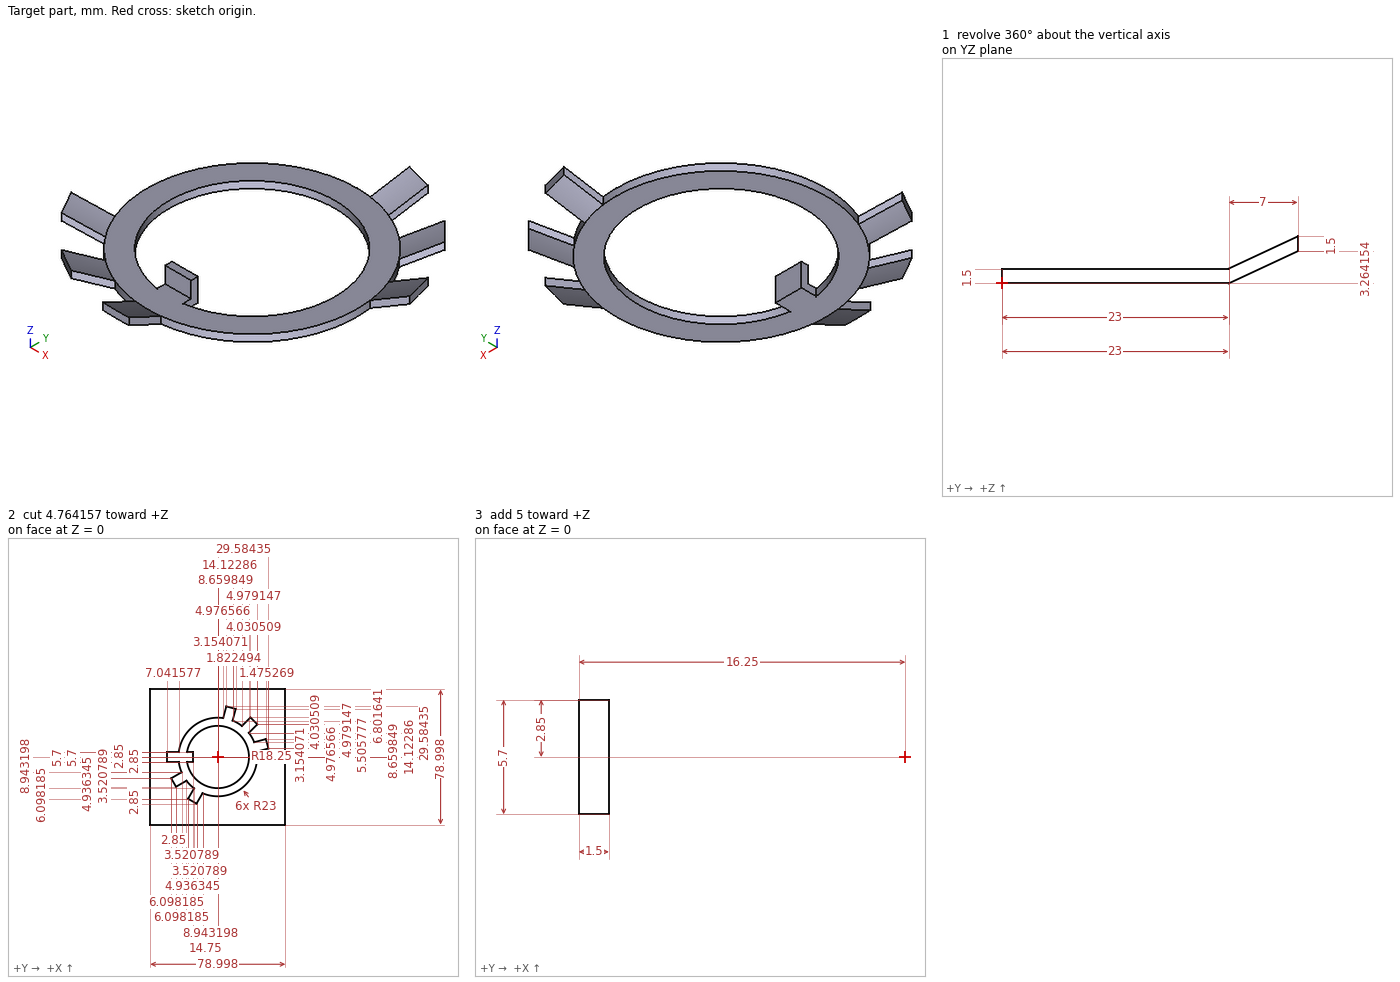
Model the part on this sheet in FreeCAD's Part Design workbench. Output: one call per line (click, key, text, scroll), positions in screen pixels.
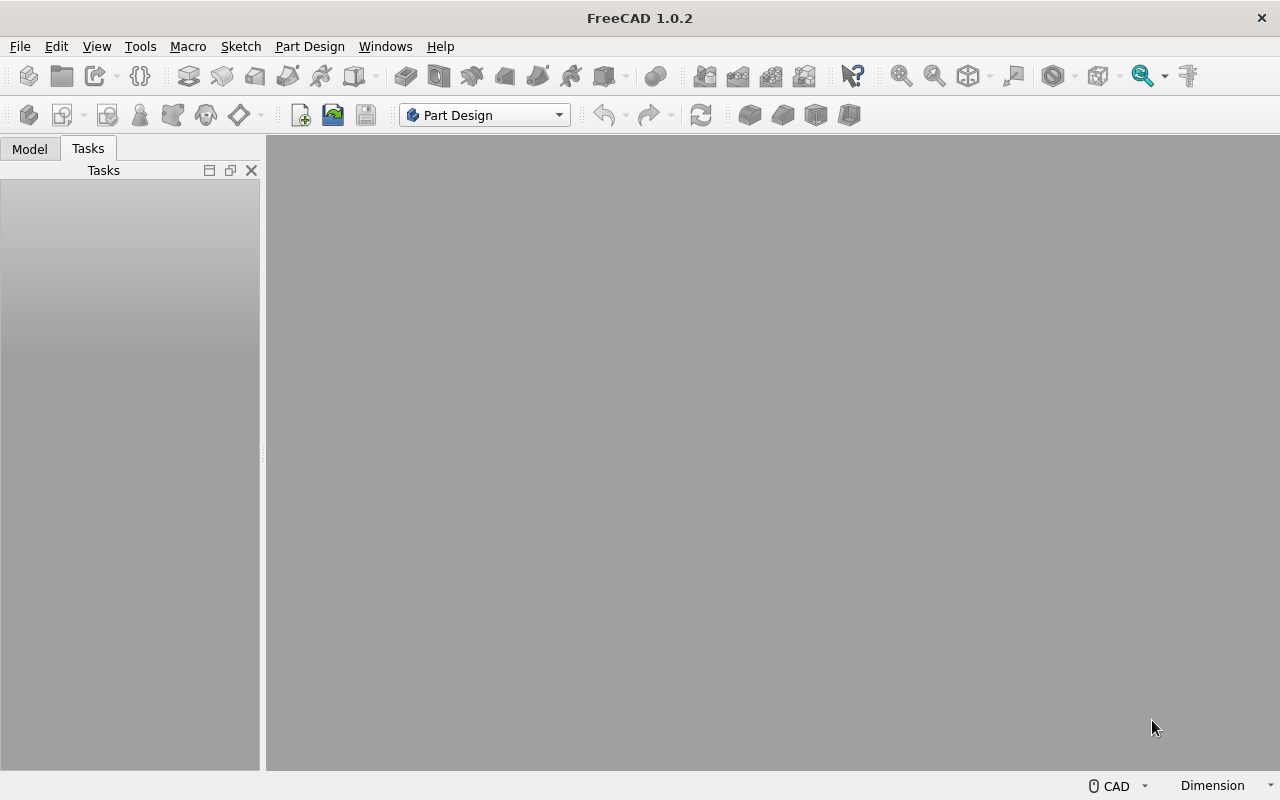
click(300, 116)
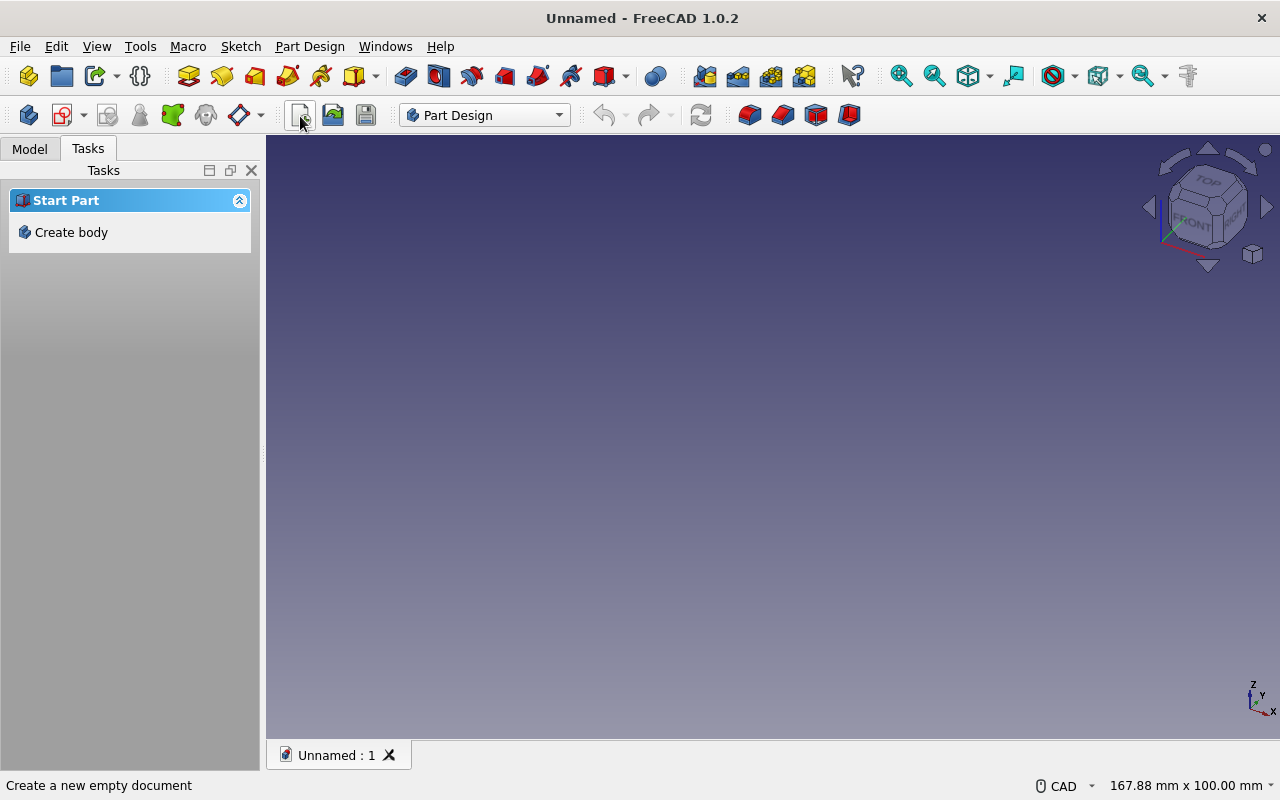
click(62, 116)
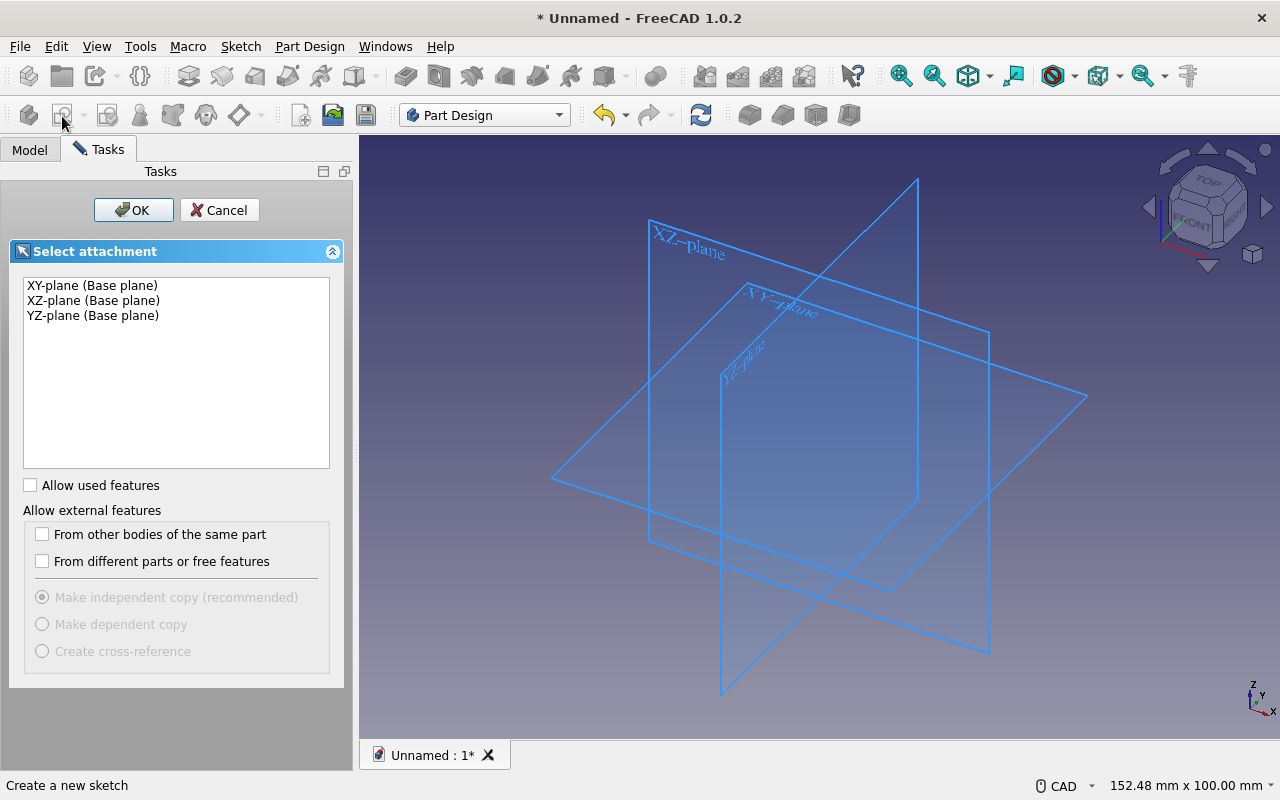
click(84, 316)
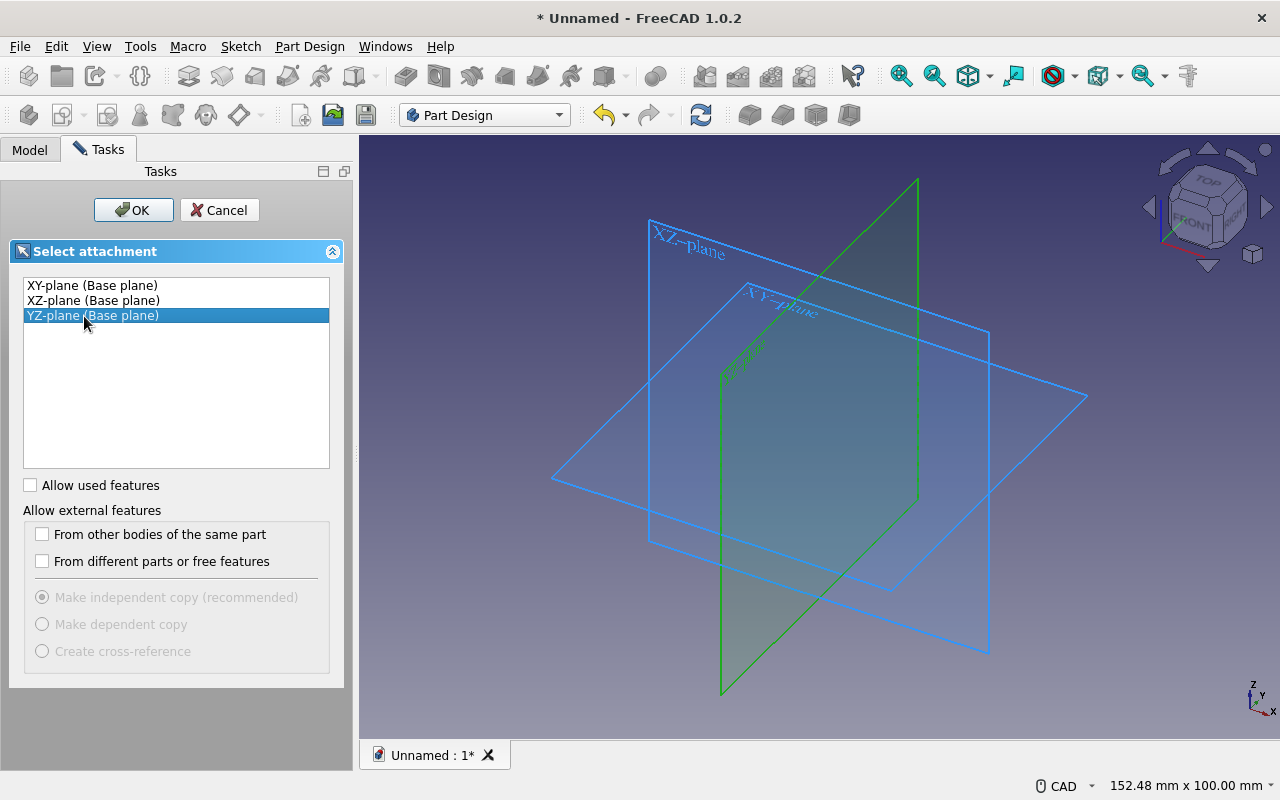
click(134, 210)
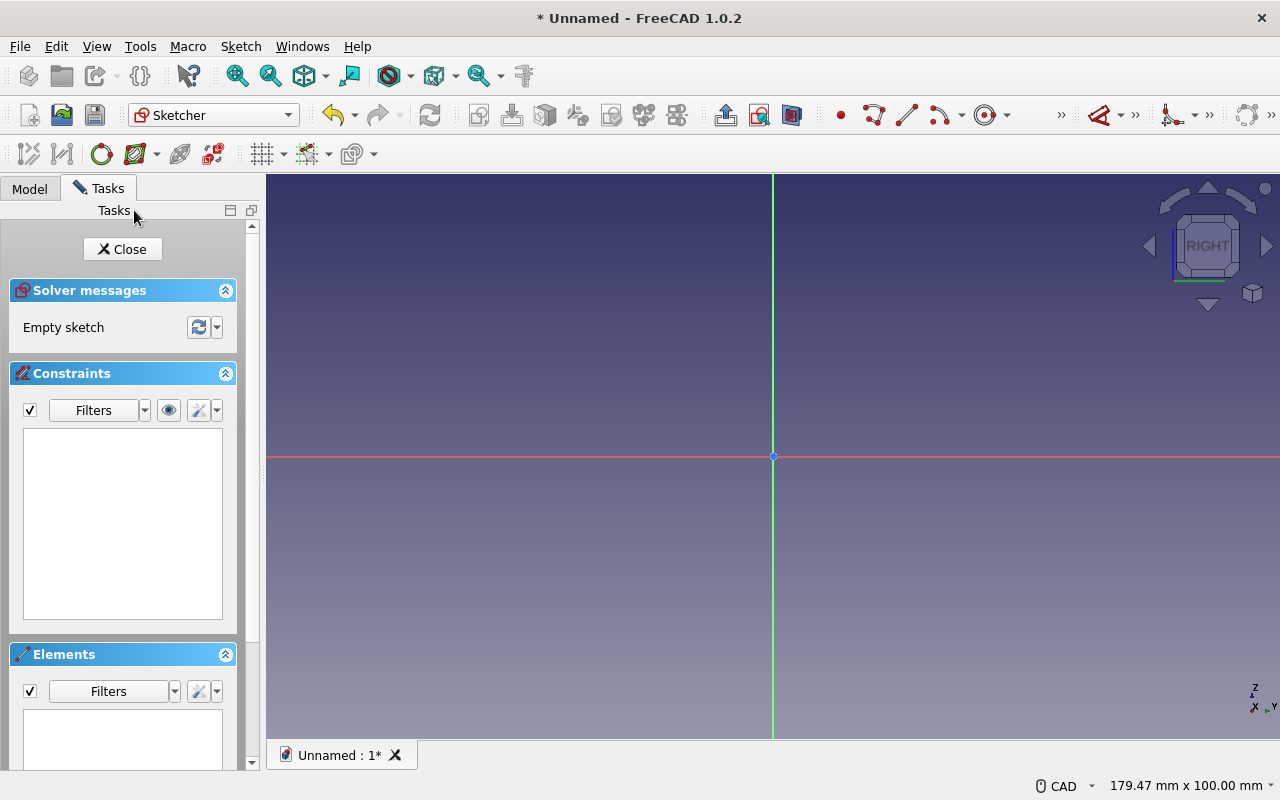
scroll(924, 437, up, 6)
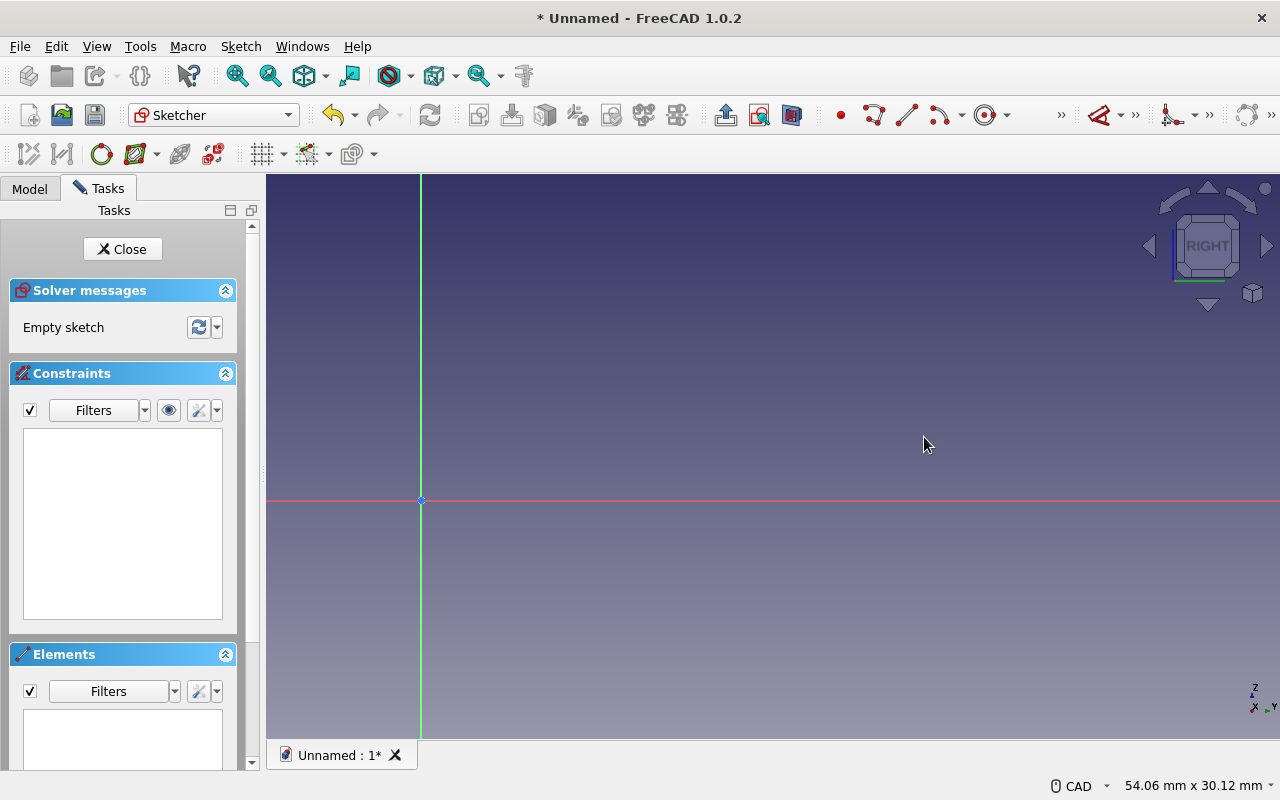
click(874, 116)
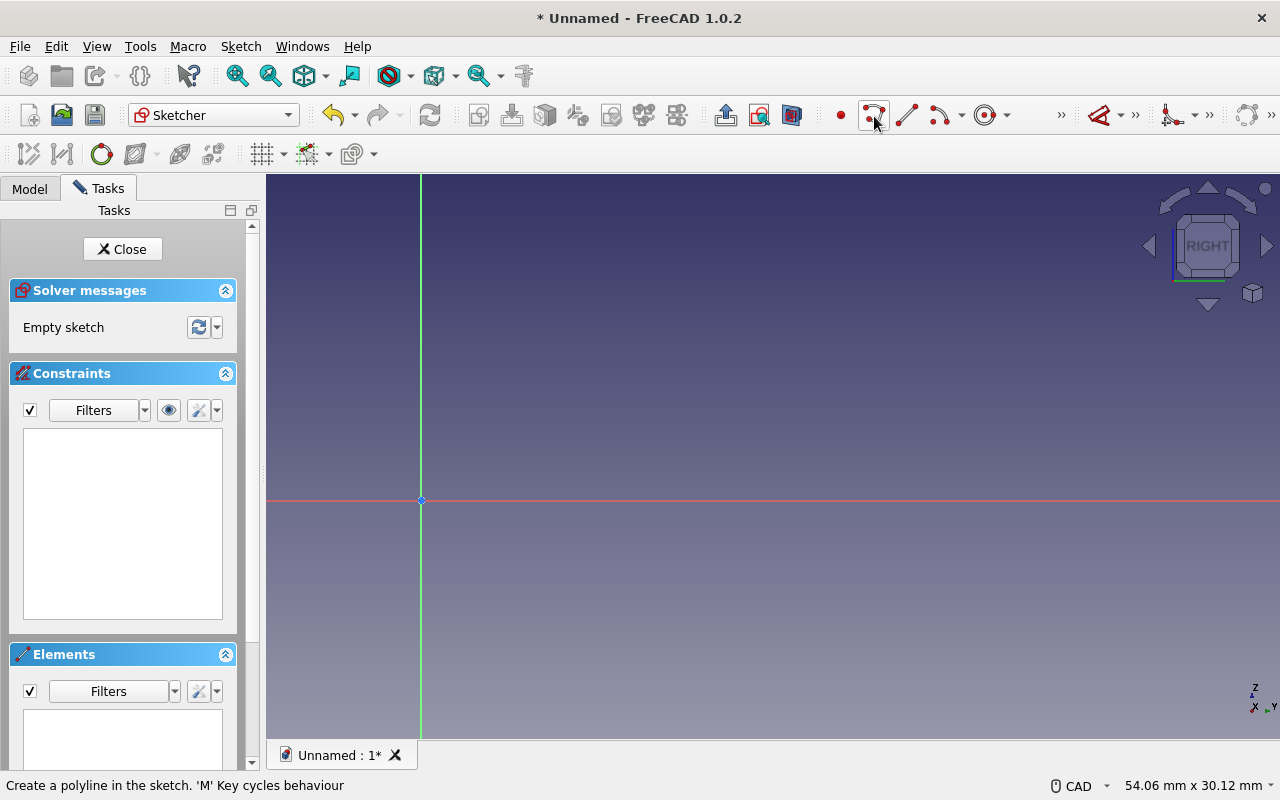
click(421, 501)
click(853, 492)
click(984, 439)
click(984, 411)
click(853, 473)
click(430, 473)
click(421, 501)
key(Escape)
key(Escape)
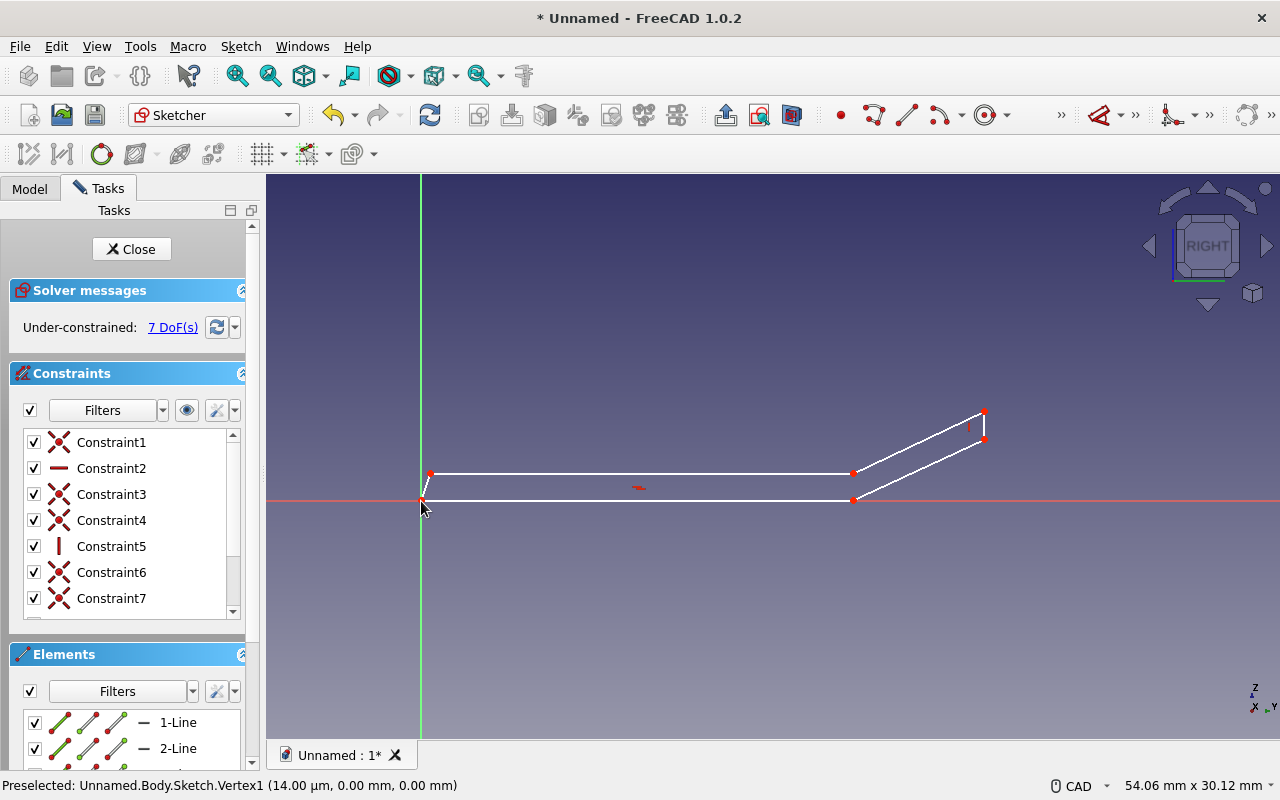
scroll(425, 490, up, 2)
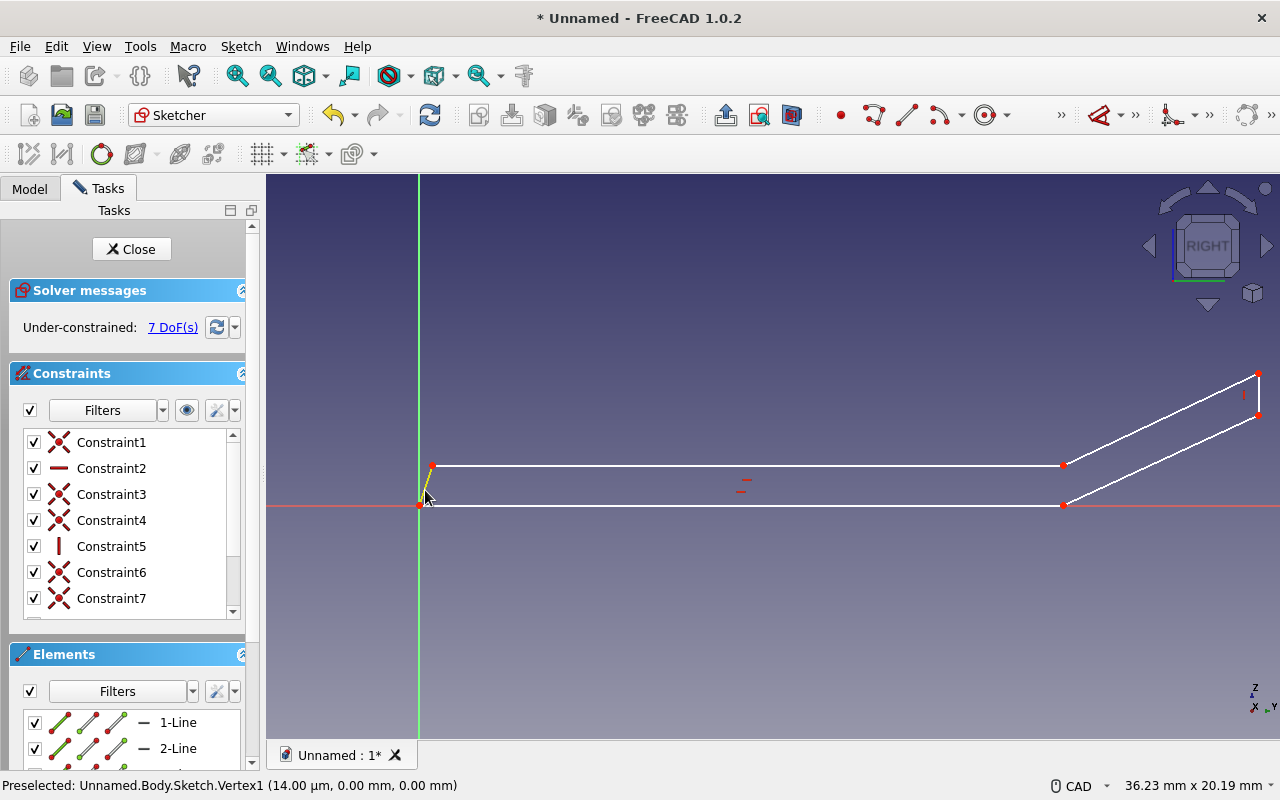
click(424, 490)